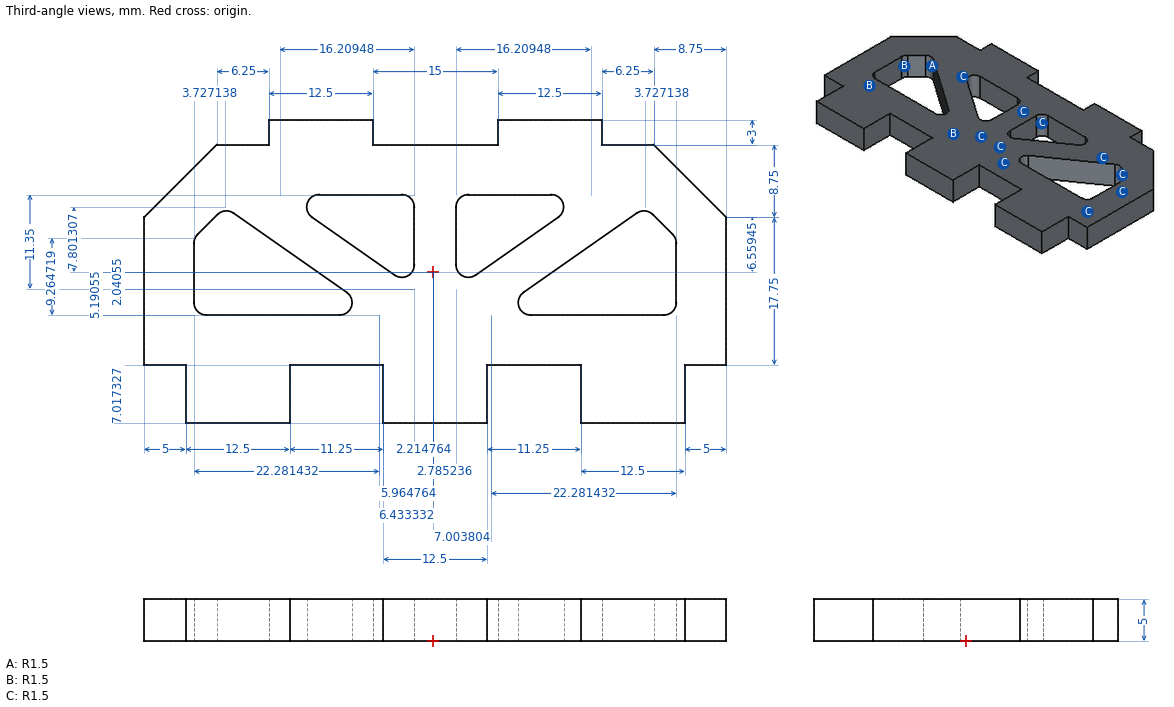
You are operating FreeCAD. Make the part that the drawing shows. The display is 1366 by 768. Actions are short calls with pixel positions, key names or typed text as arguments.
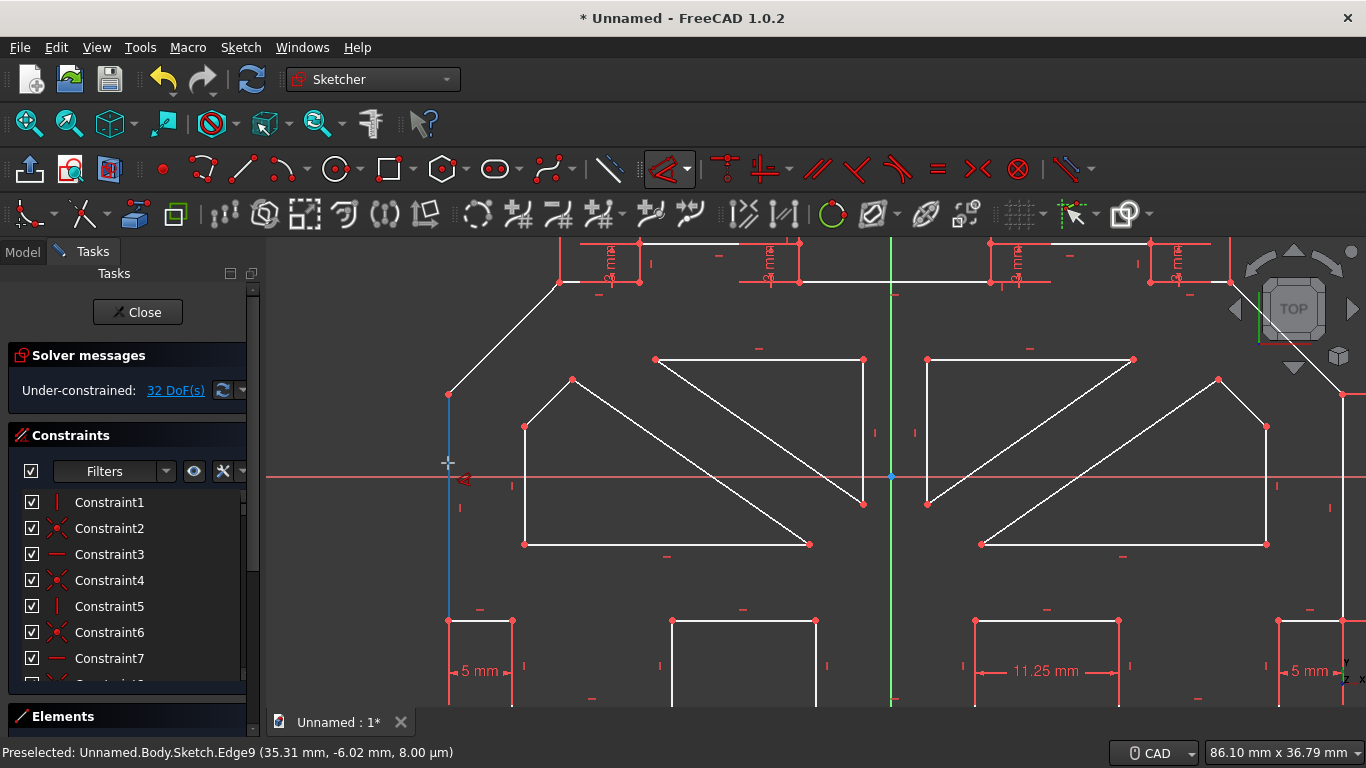
click(449, 462)
click(415, 508)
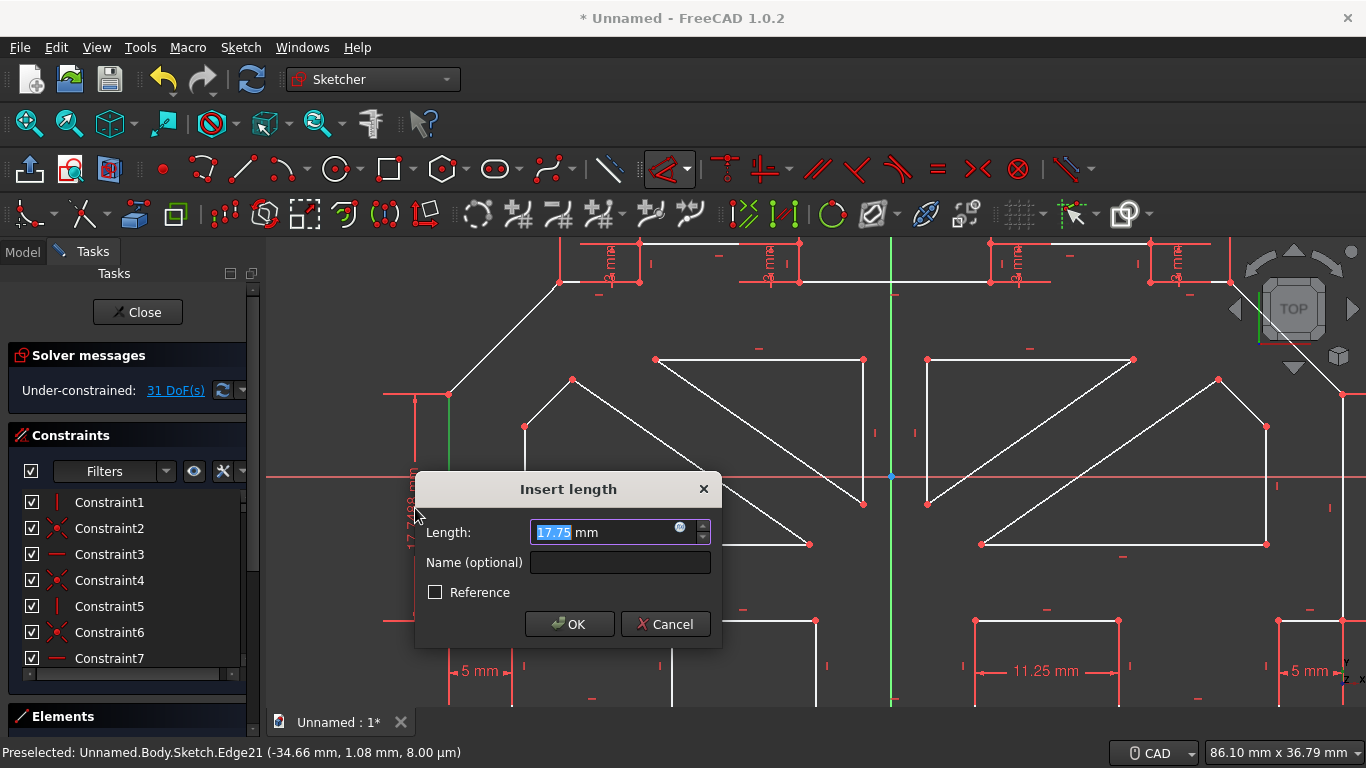
text(17.75)
key(Return)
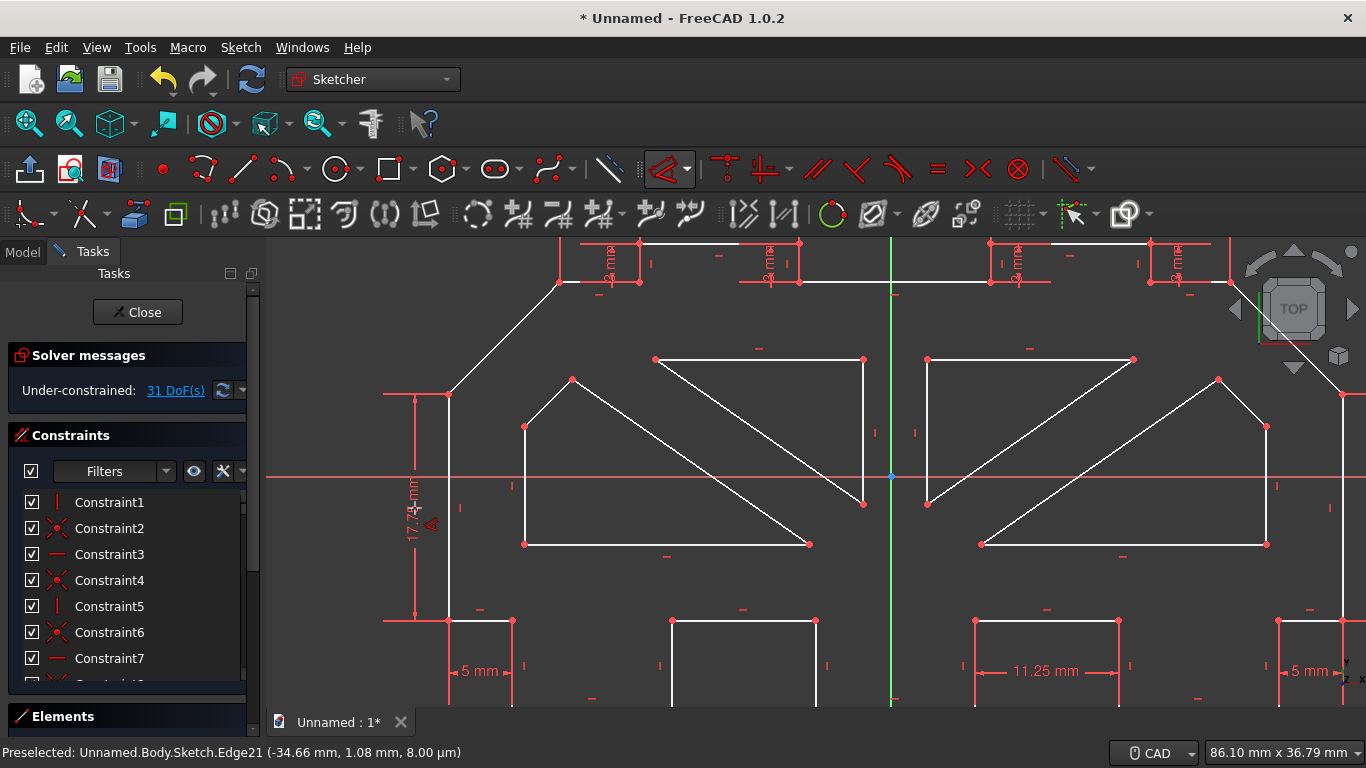
click(715, 621)
click(744, 655)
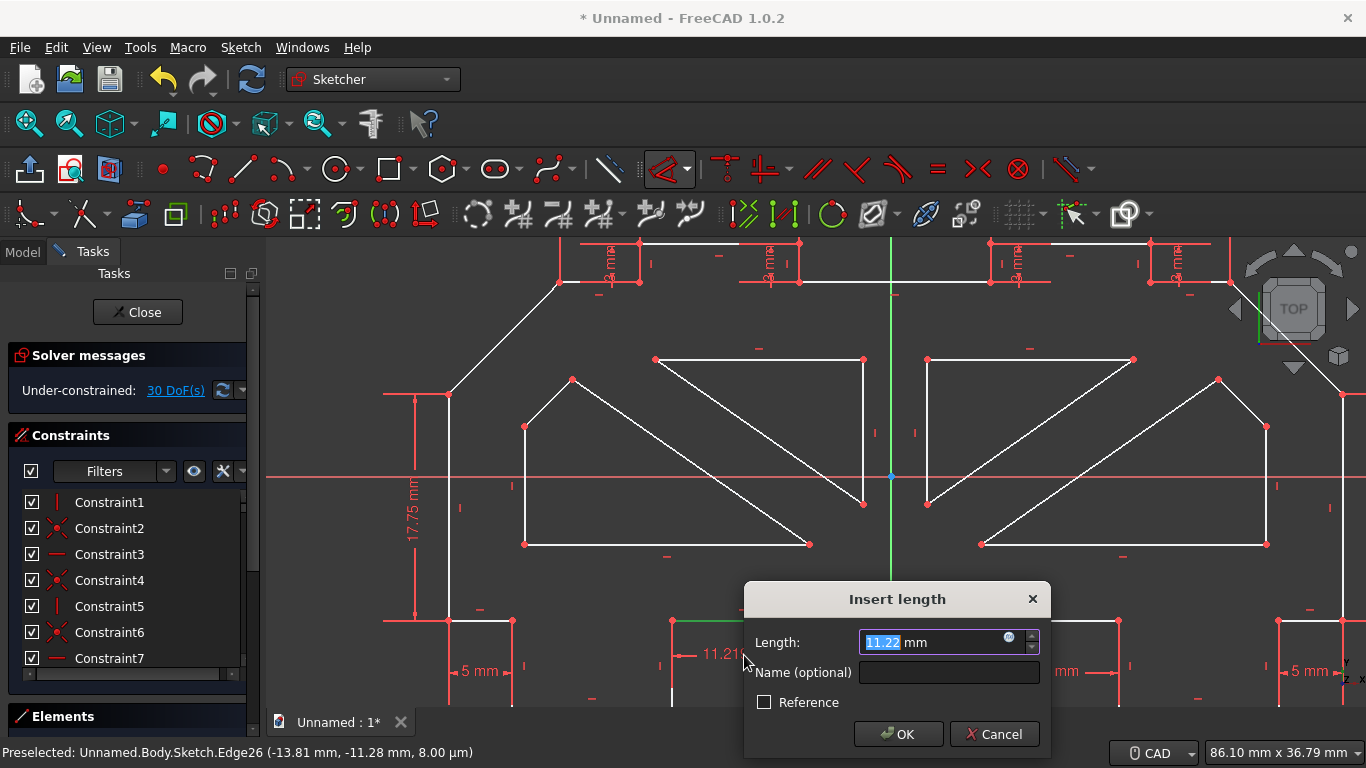
text(11.25)
key(Return)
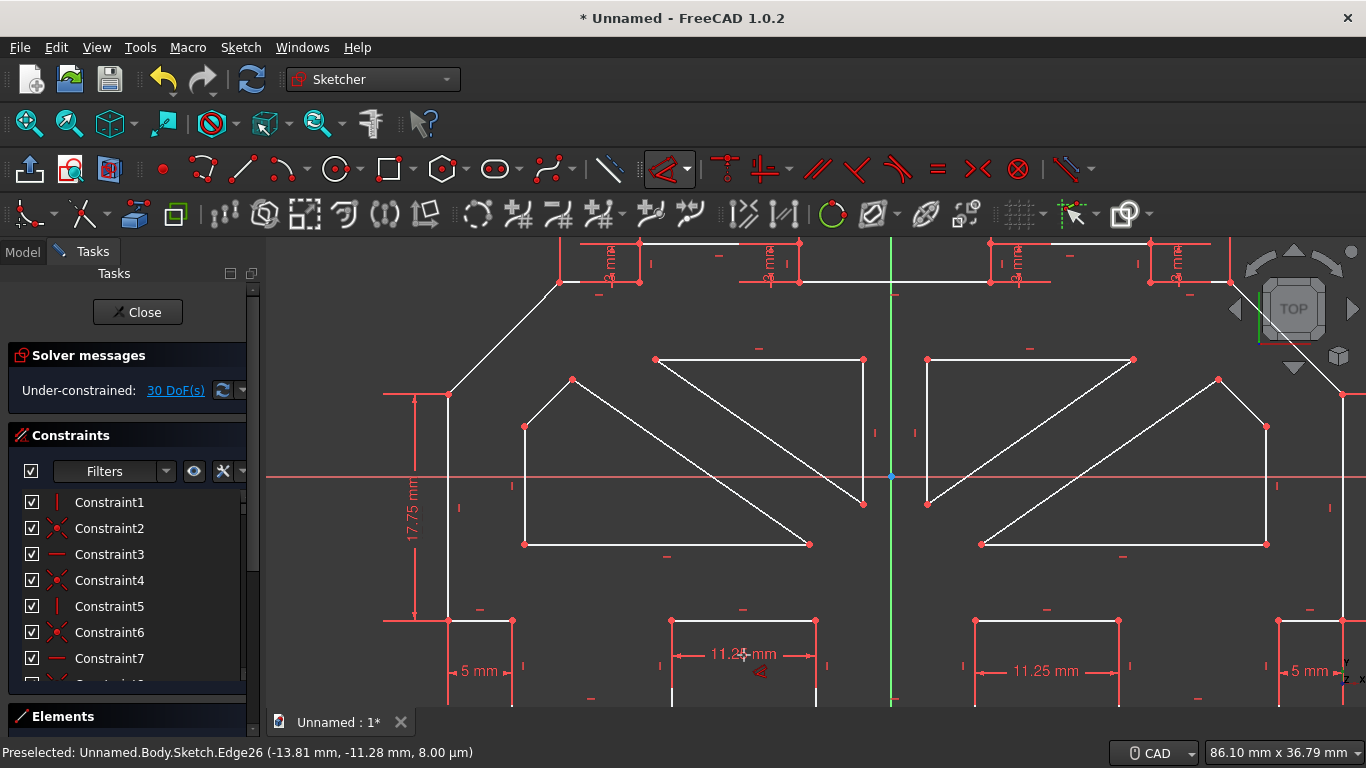
click(863, 403)
click(829, 432)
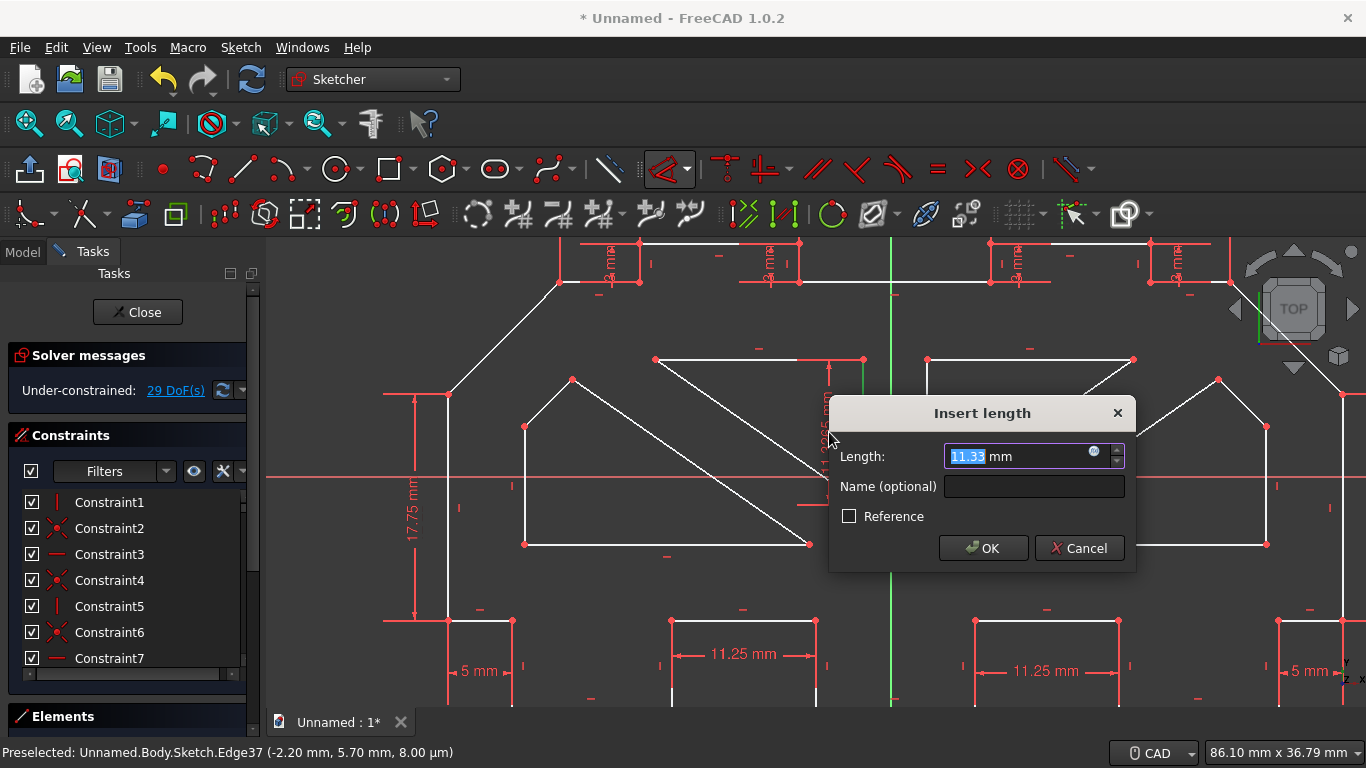
text(11.35)
key(Return)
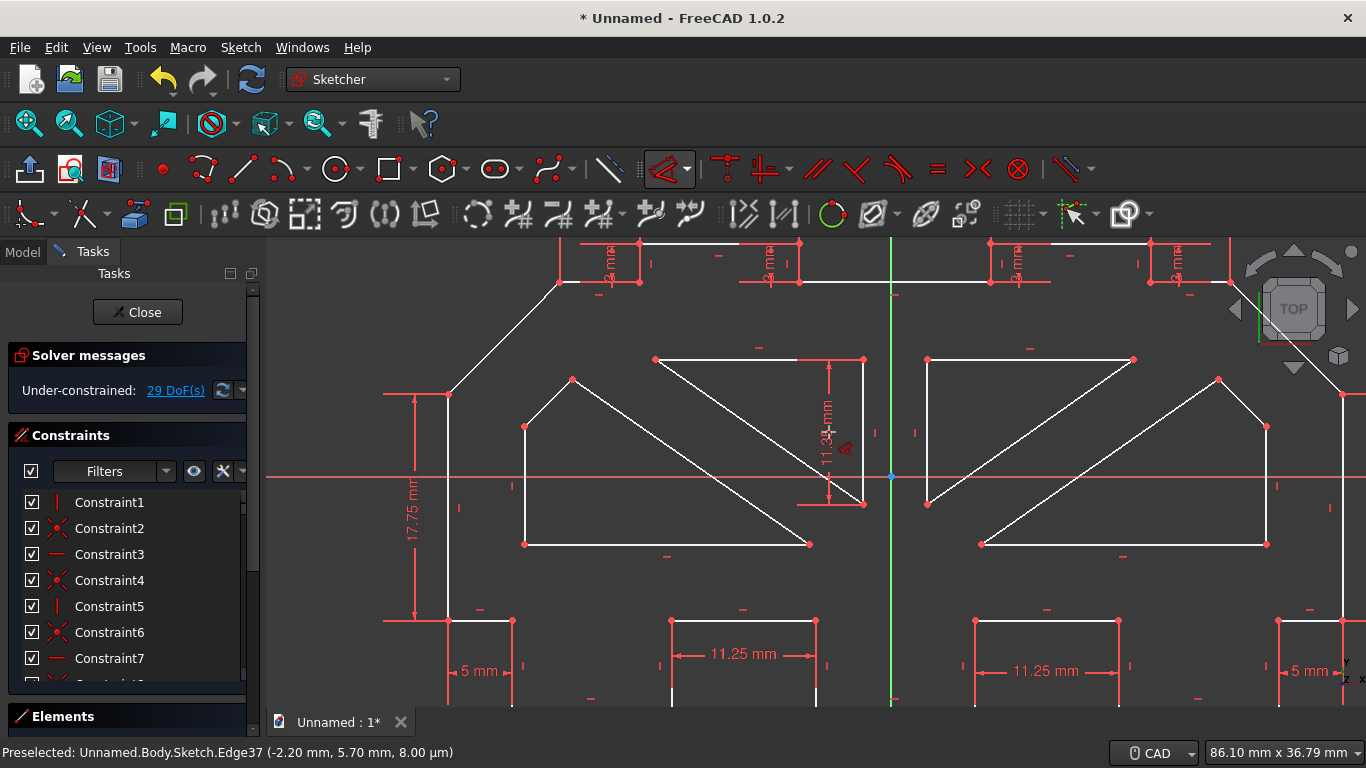
click(927, 461)
click(961, 432)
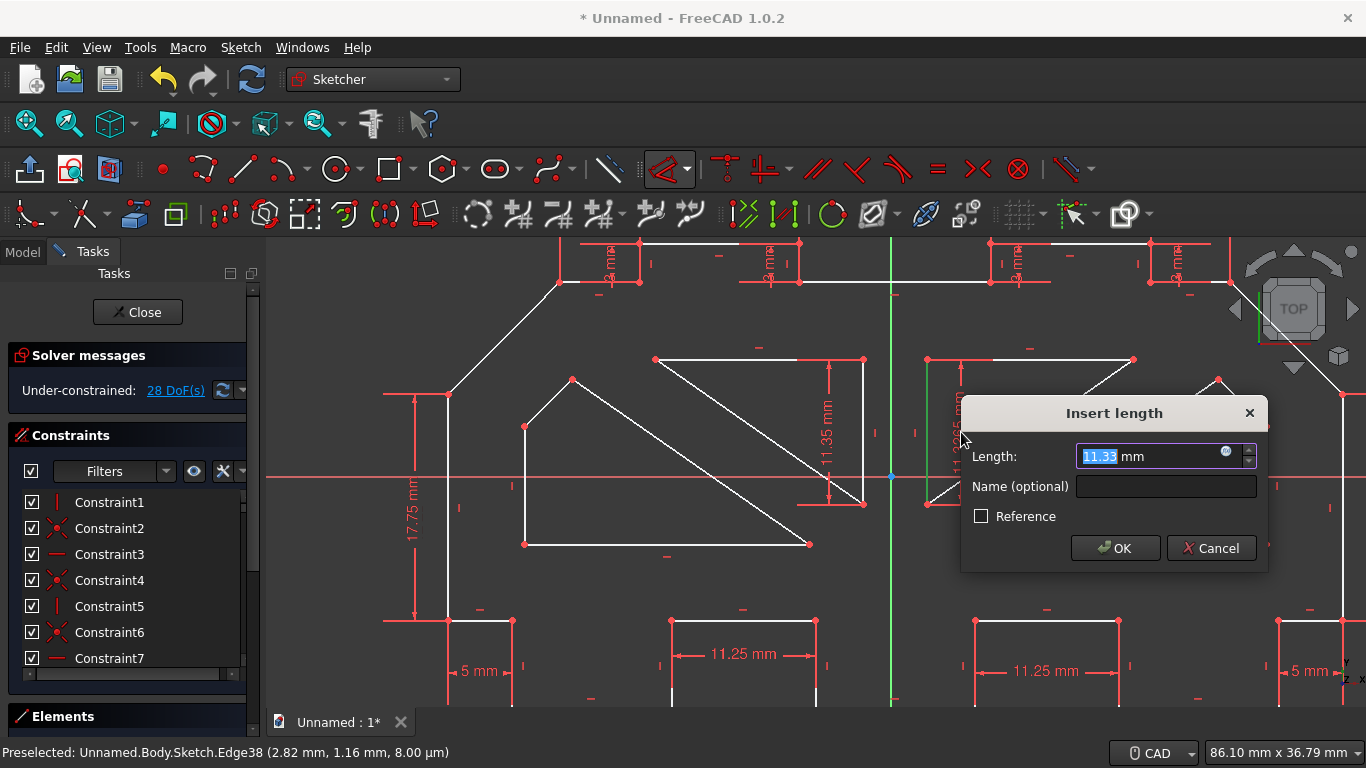
text(11.35)
key(Return)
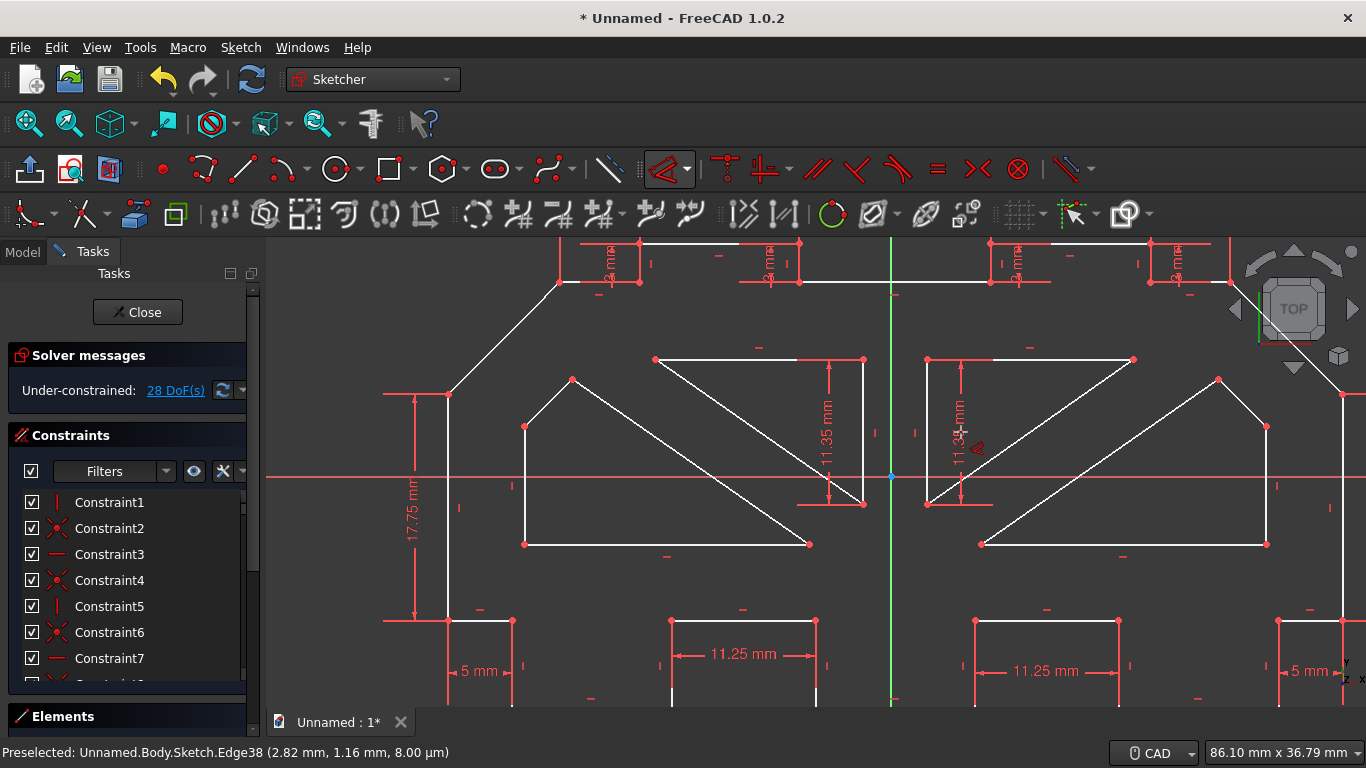
scroll(448, 464, down, 2)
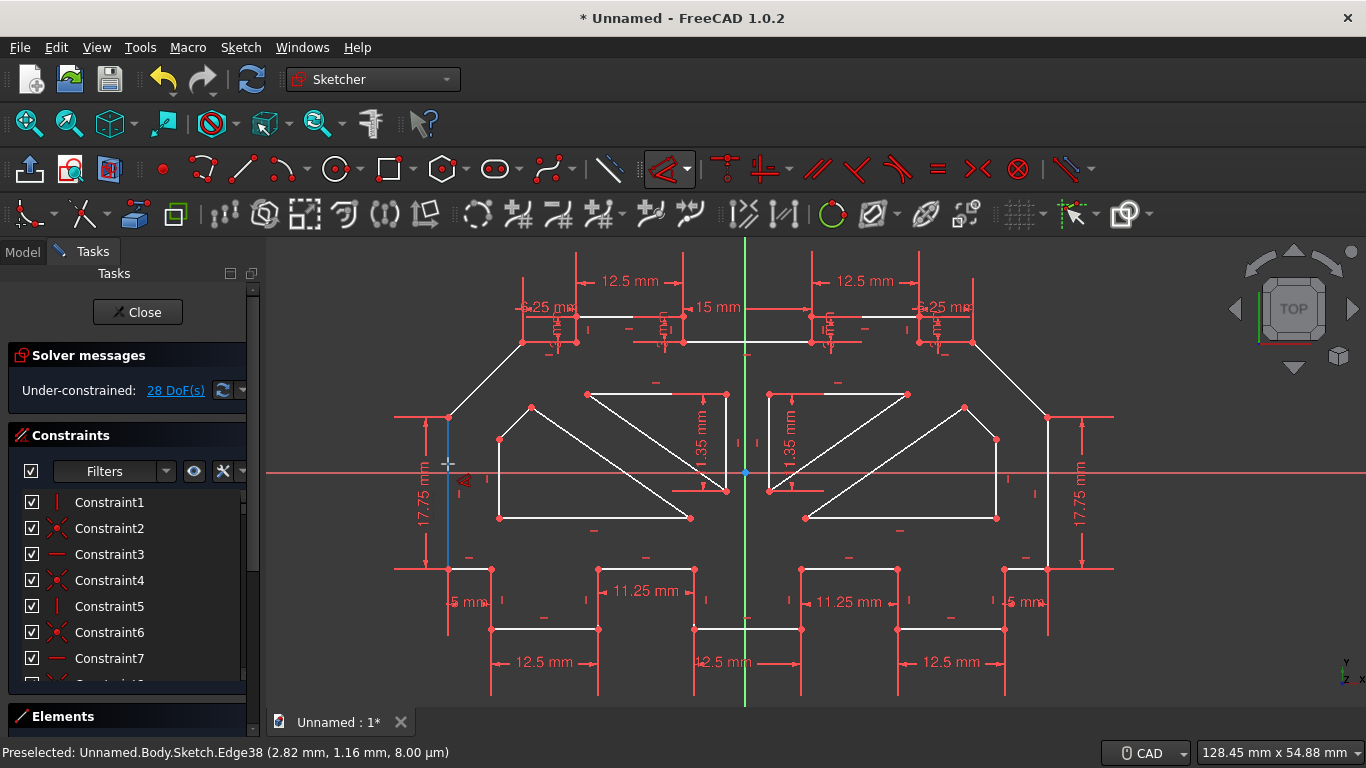
click(1025, 395)
click(1027, 308)